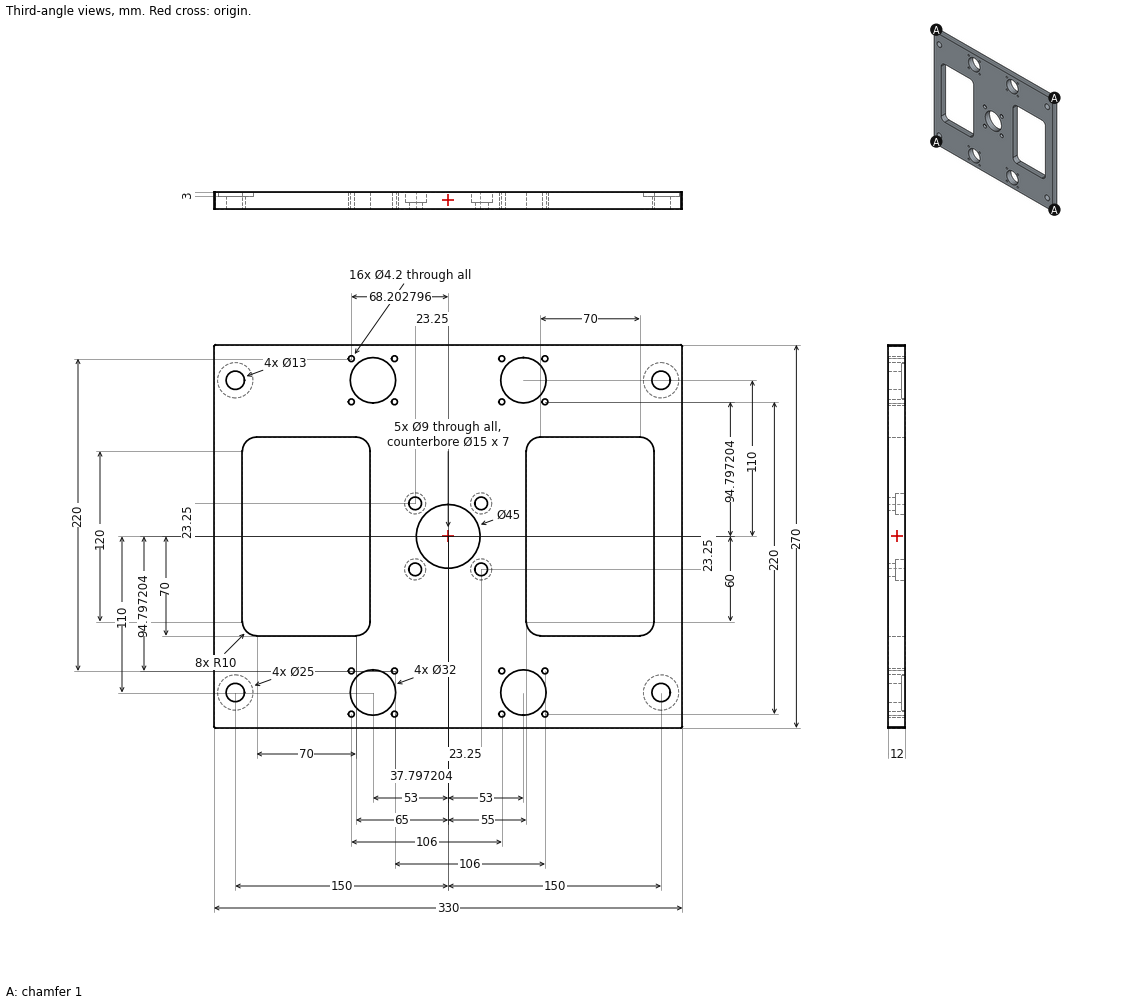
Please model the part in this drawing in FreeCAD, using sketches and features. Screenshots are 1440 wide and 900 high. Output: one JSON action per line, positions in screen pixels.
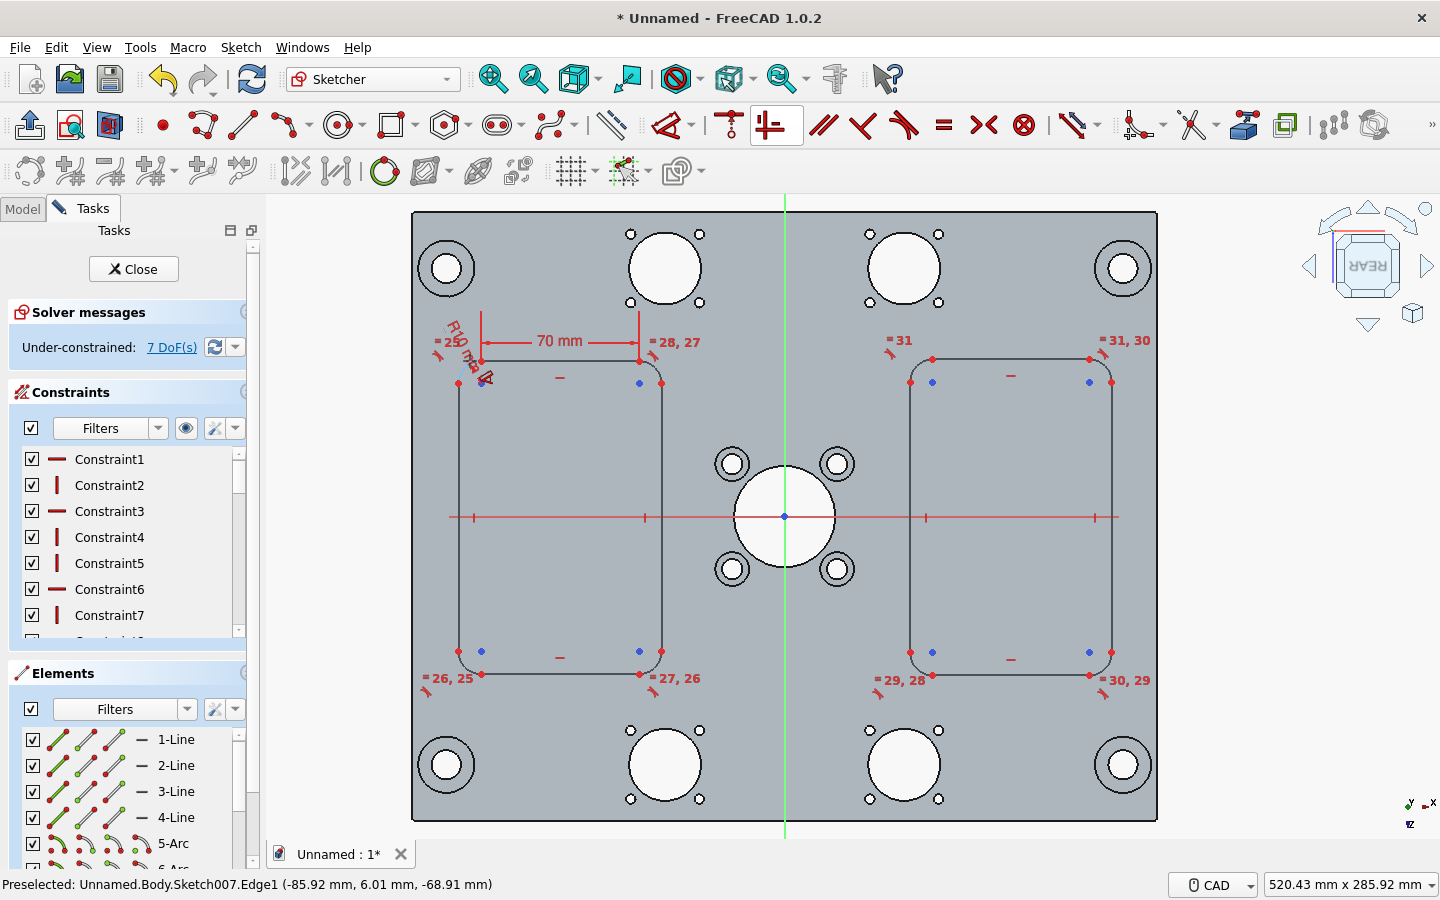
{"action": "left_click", "coordinate": [980, 675]}
{"action": "left_click", "coordinate": [1011, 709]}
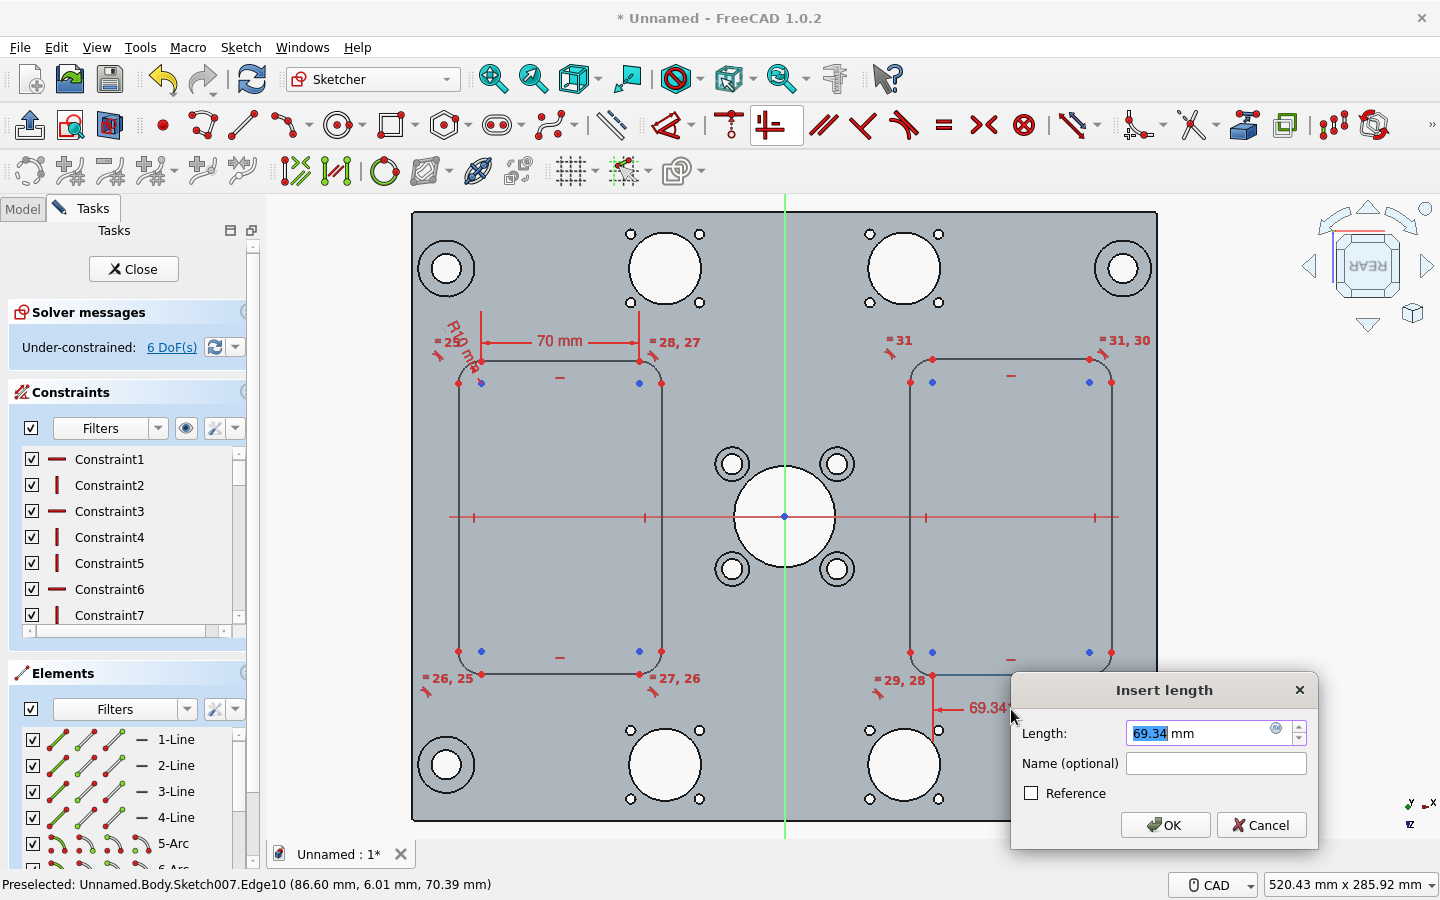
{"action": "type", "text": "70"}
{"action": "key", "text": "Return"}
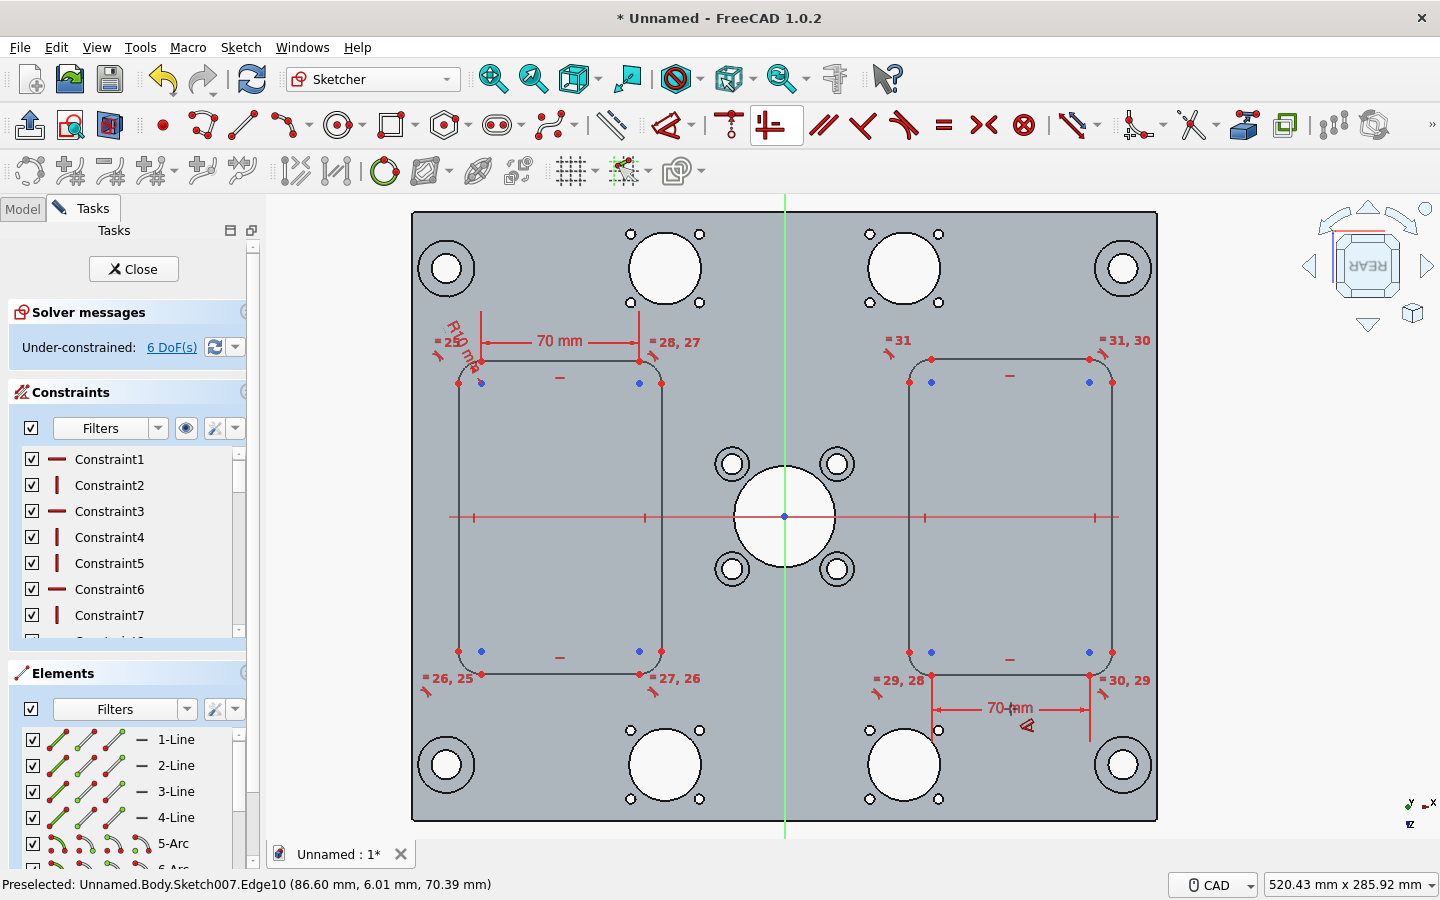
{"action": "left_click", "coordinate": [459, 464]}
{"action": "left_click", "coordinate": [425, 456]}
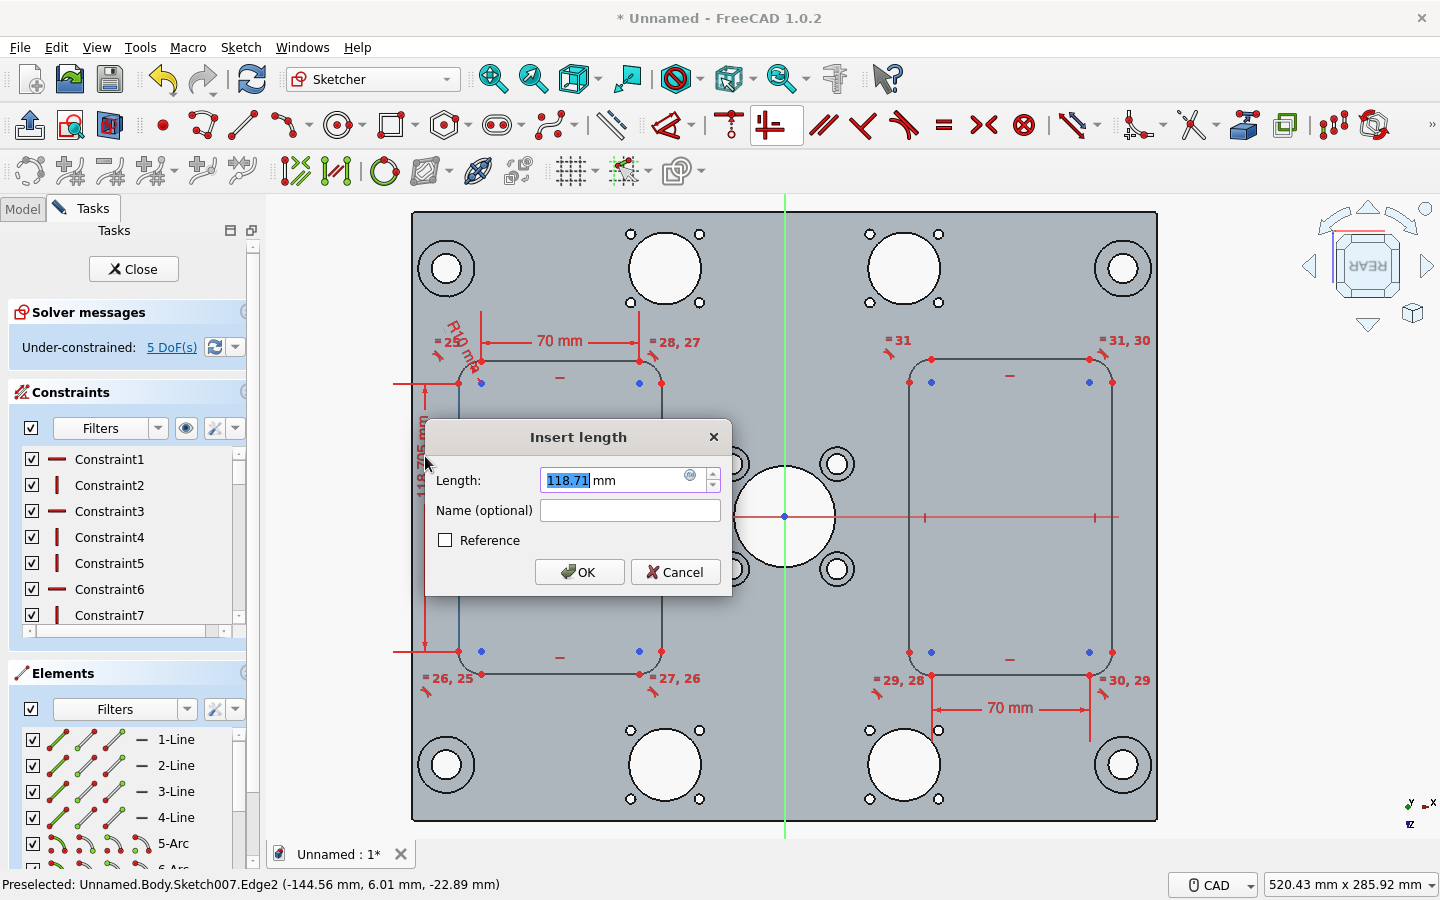
{"action": "type", "text": "120"}
{"action": "key", "text": "Return"}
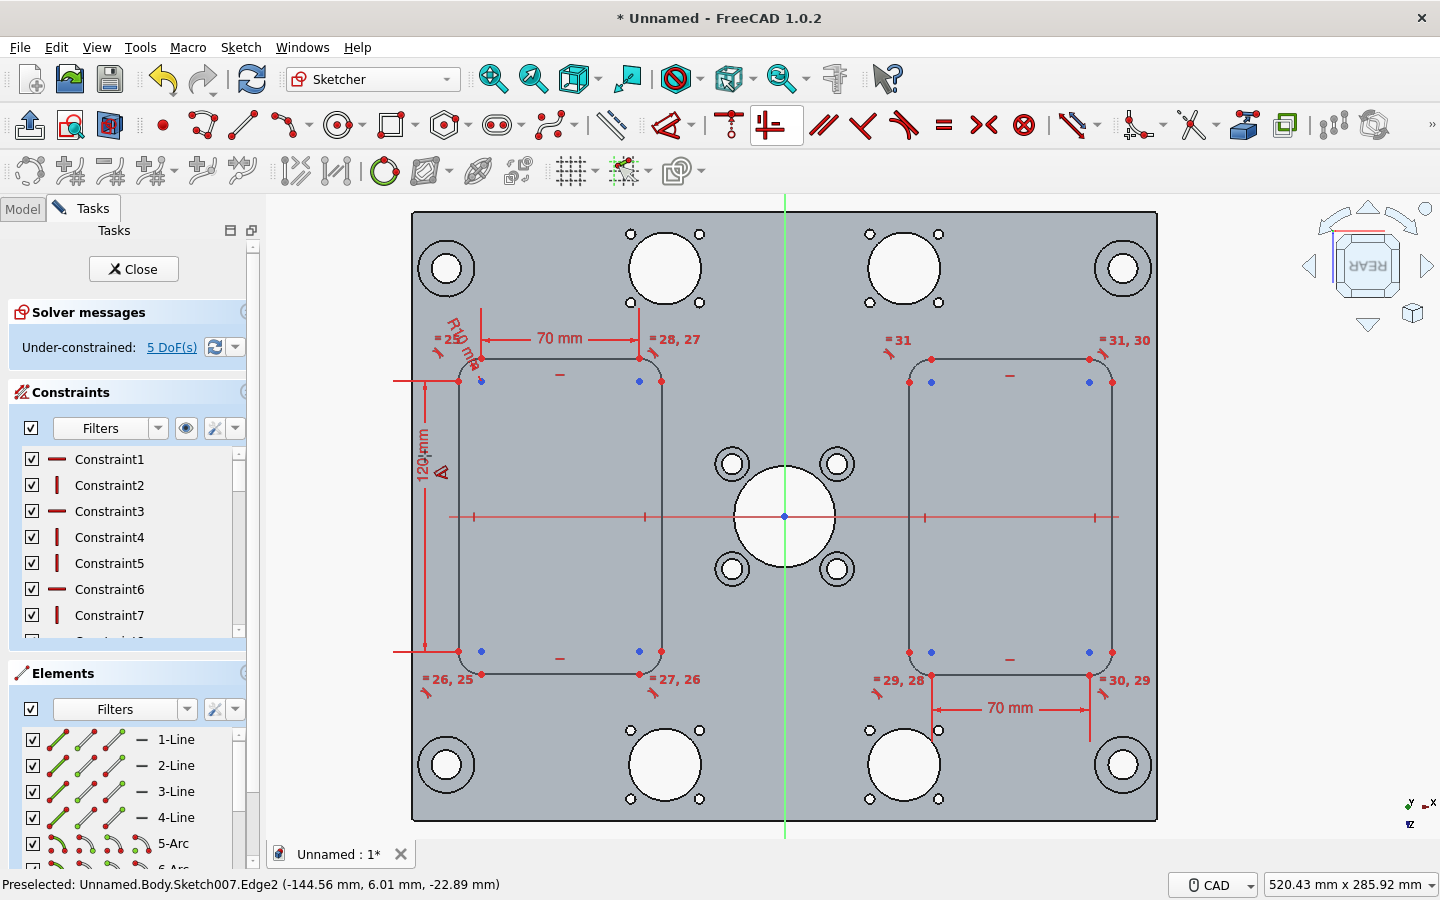
{"action": "left_click", "coordinate": [909, 463]}
{"action": "left_click", "coordinate": [943, 455]}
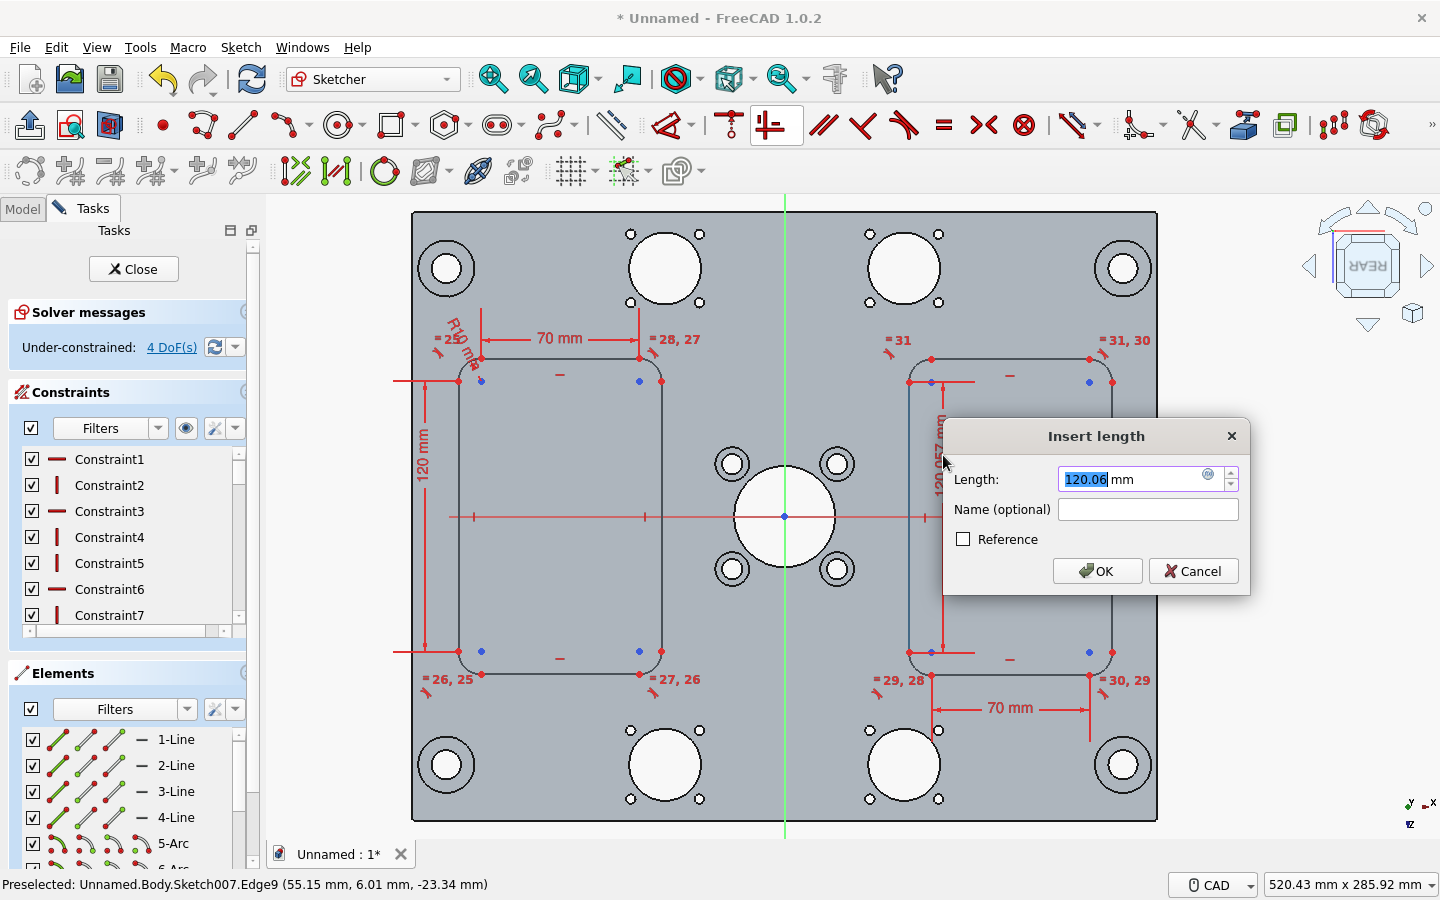
{"action": "type", "text": "120"}
{"action": "key", "text": "Return"}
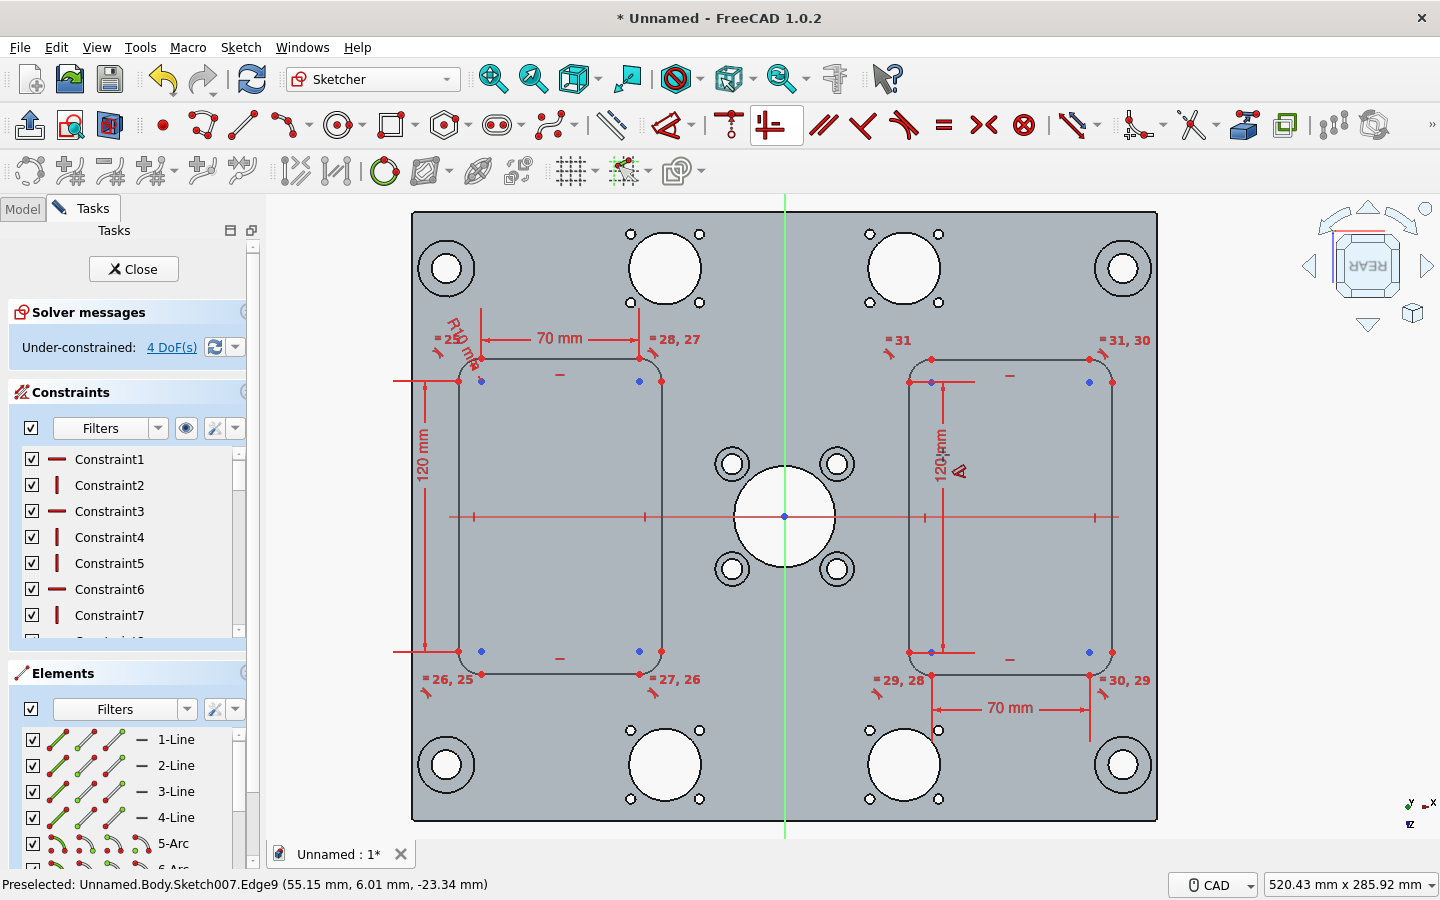
{"action": "left_click", "coordinate": [639, 359]}
{"action": "left_click", "coordinate": [712, 325]}